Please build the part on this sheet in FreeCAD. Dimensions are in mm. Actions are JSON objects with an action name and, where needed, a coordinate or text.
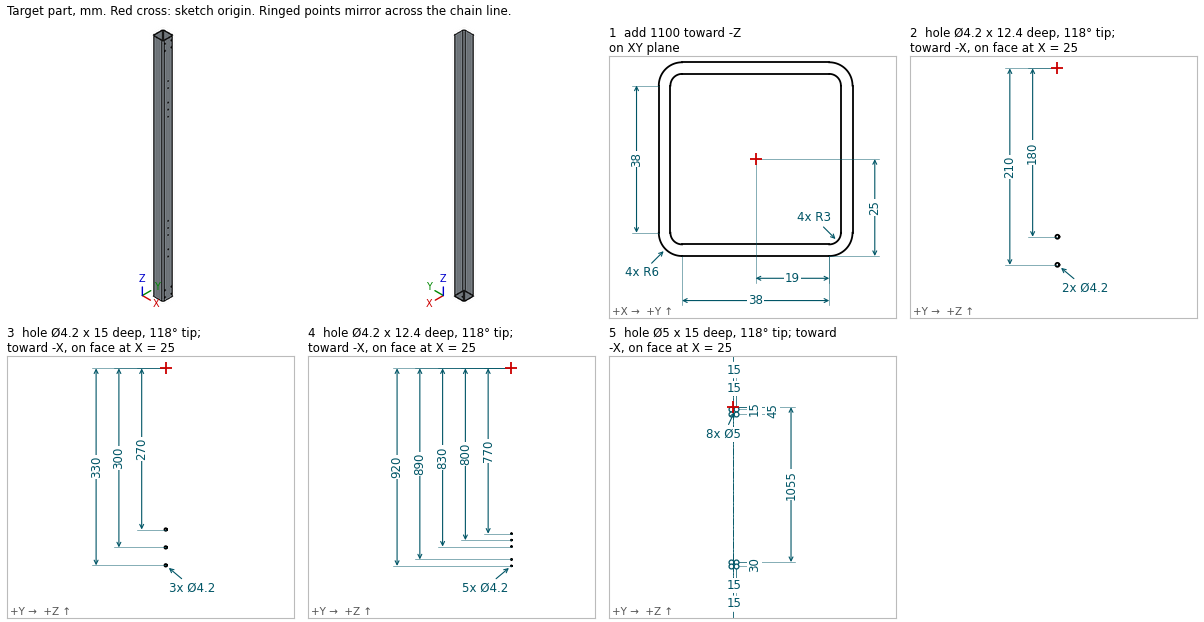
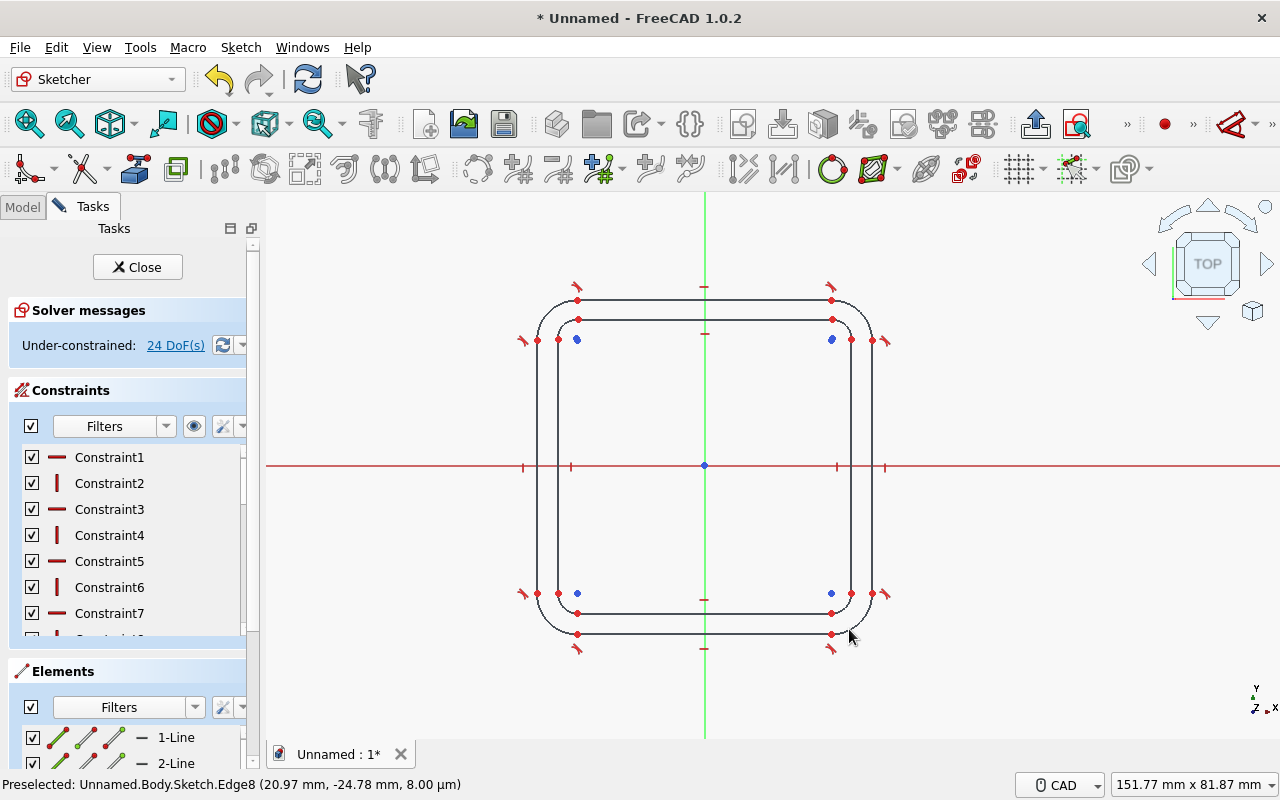
{"action": "left_click", "coordinate": [654, 614]}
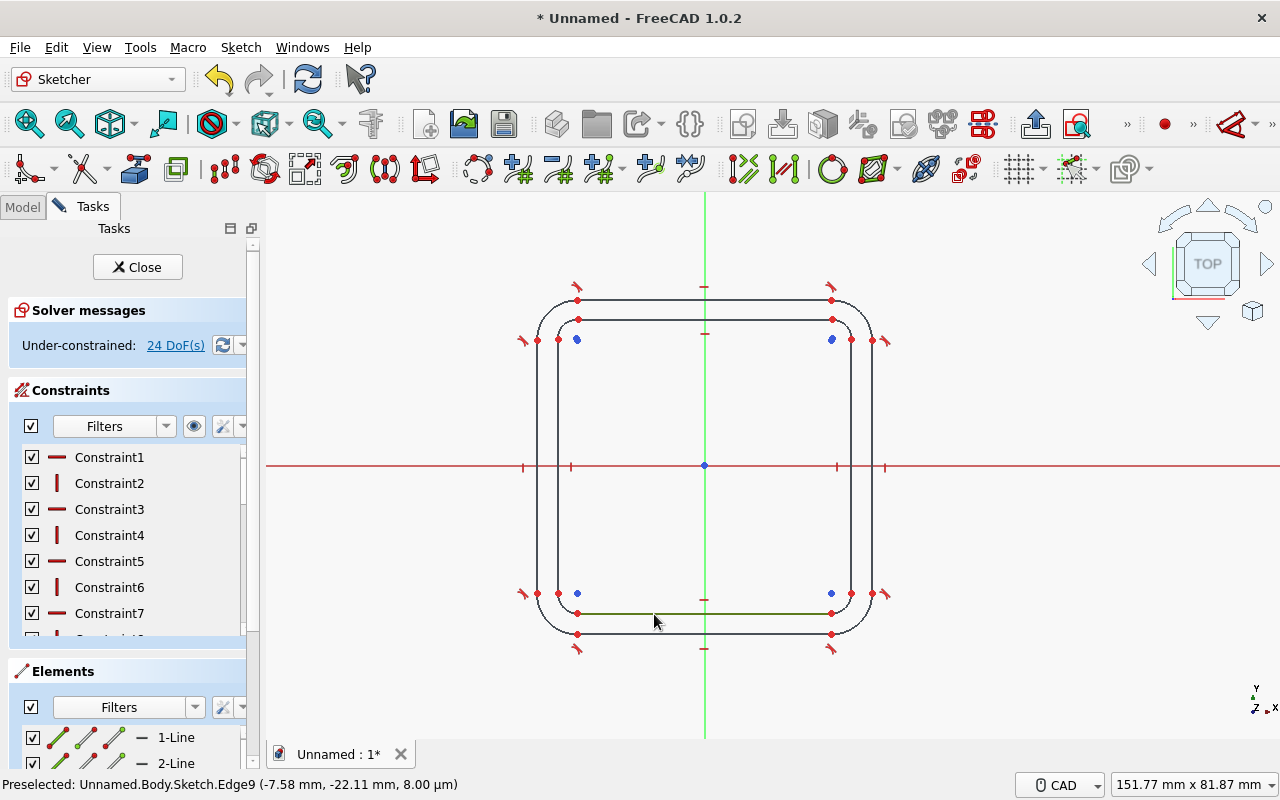
{"action": "scroll", "coordinate": [840, 611], "scroll_direction": "up", "scroll_amount": 2}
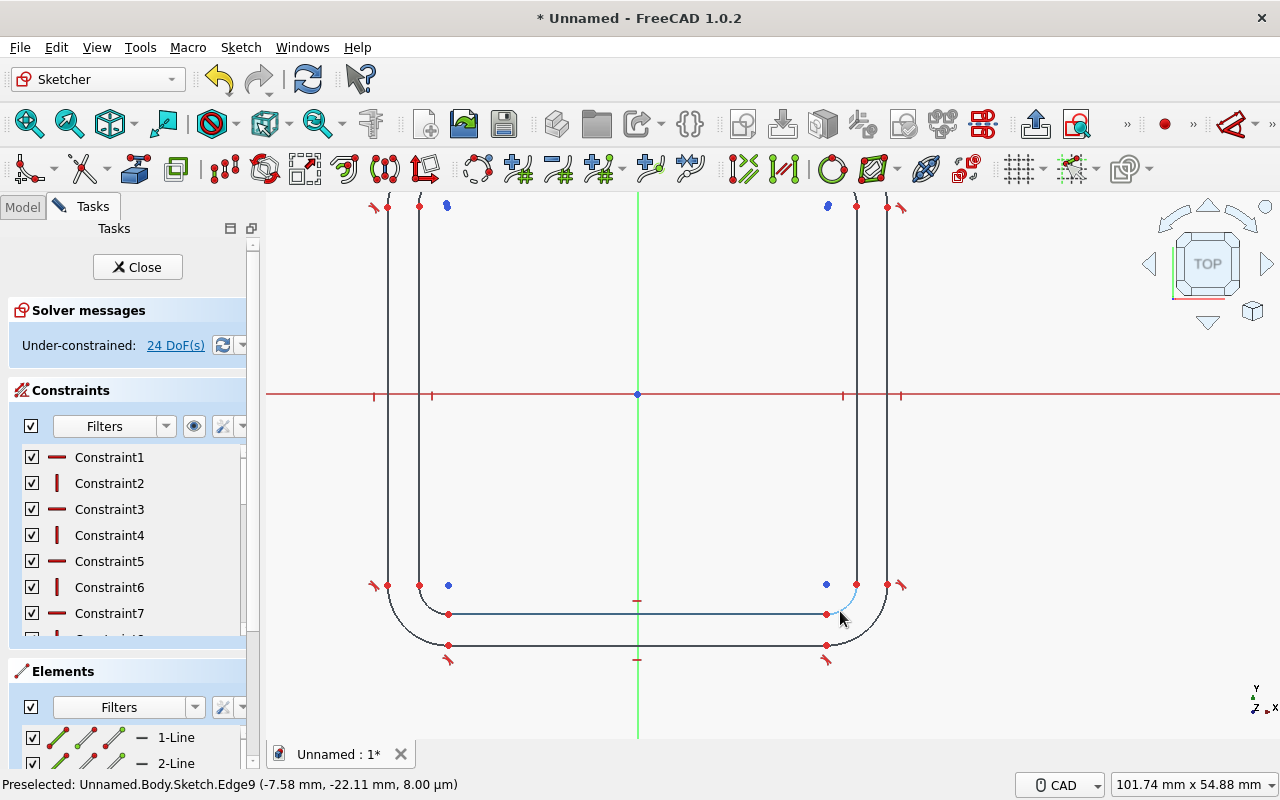
{"action": "left_click", "coordinate": [840, 611]}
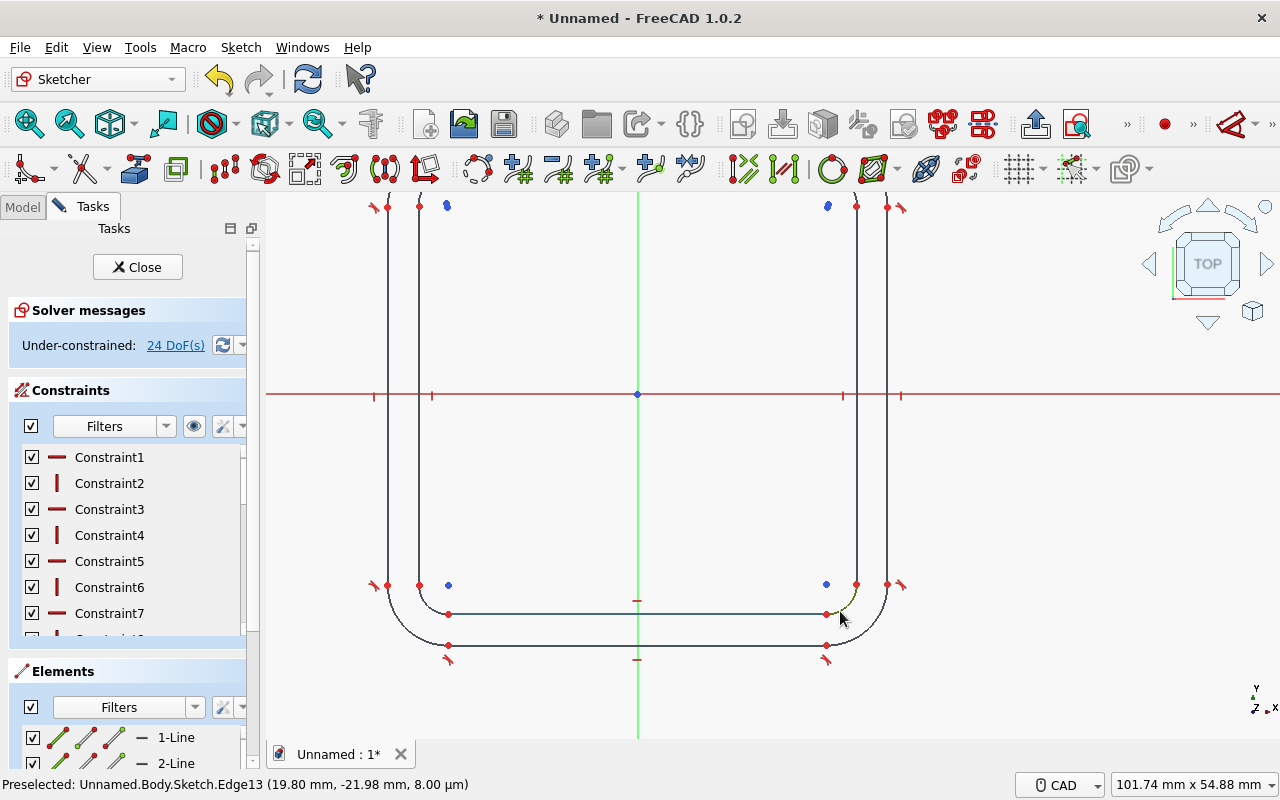
{"action": "key", "text": "t"}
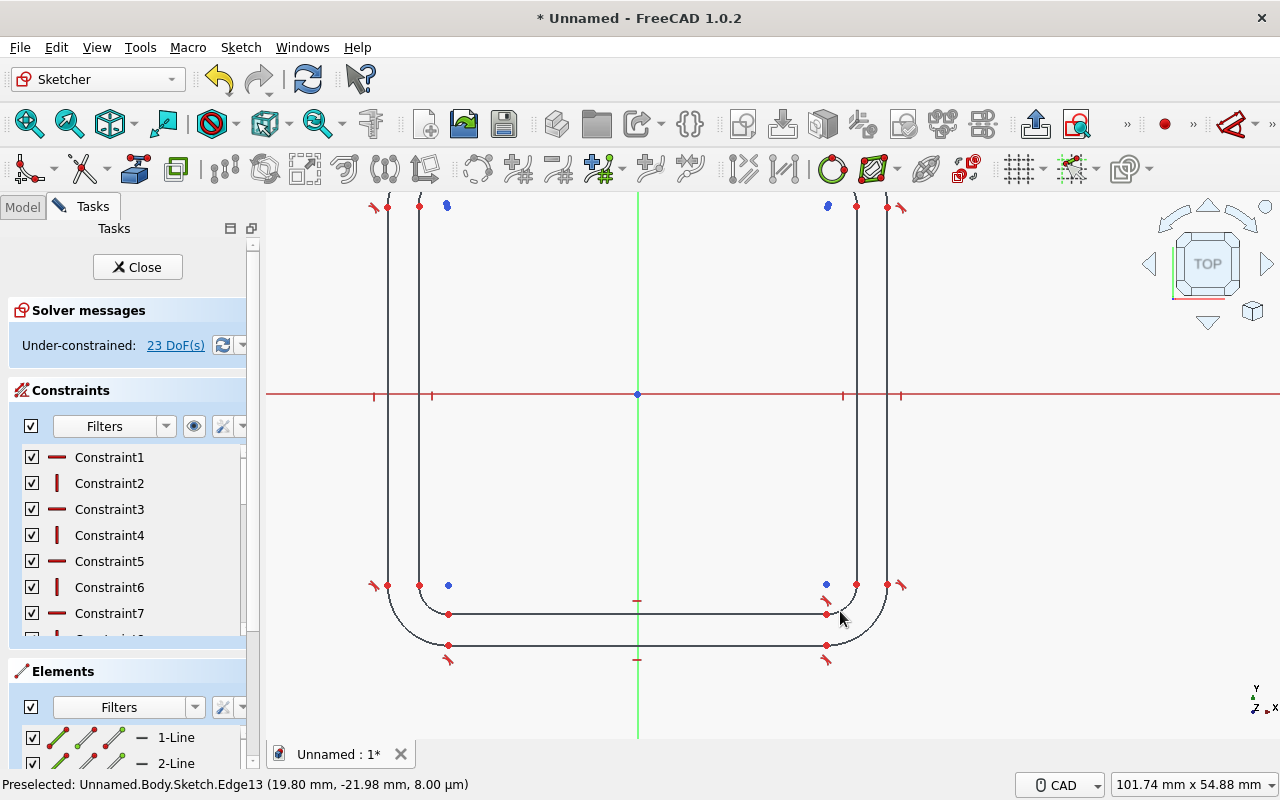
{"action": "left_click", "coordinate": [562, 614]}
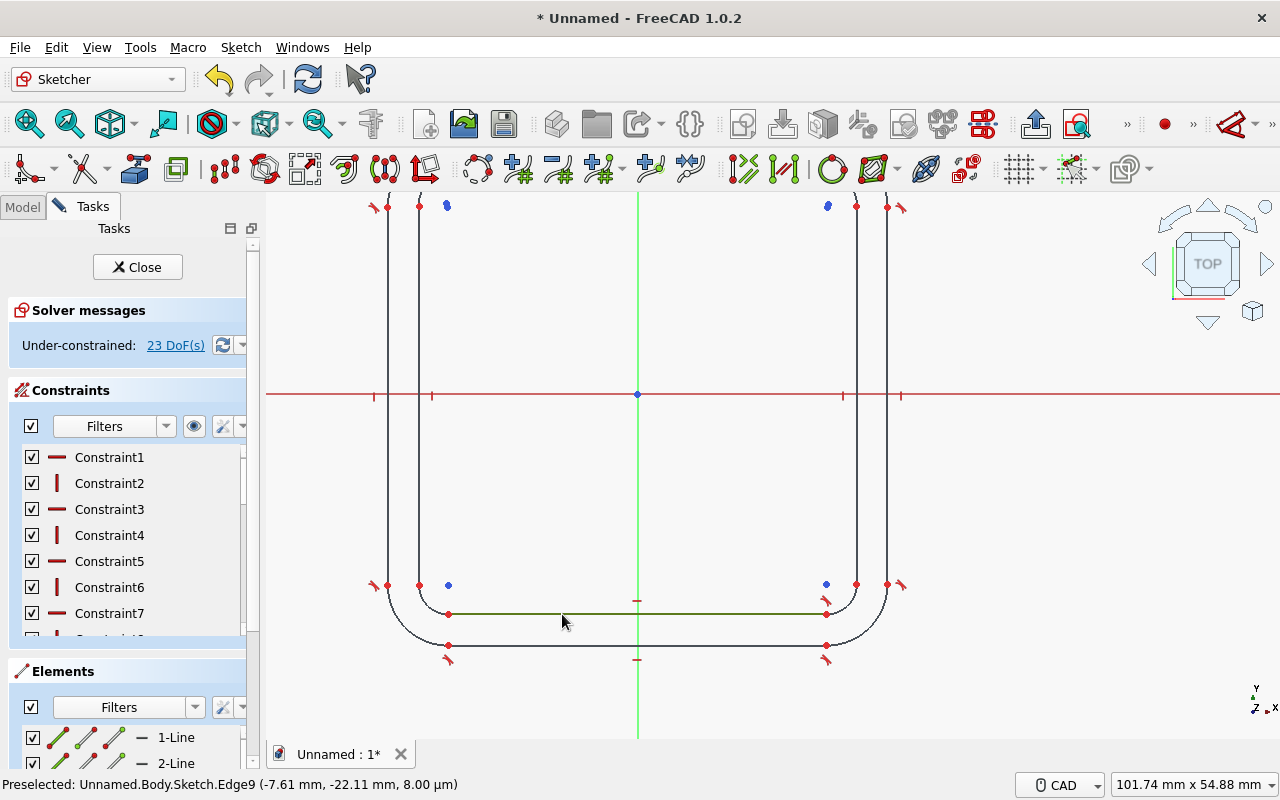
{"action": "left_click", "coordinate": [422, 599]}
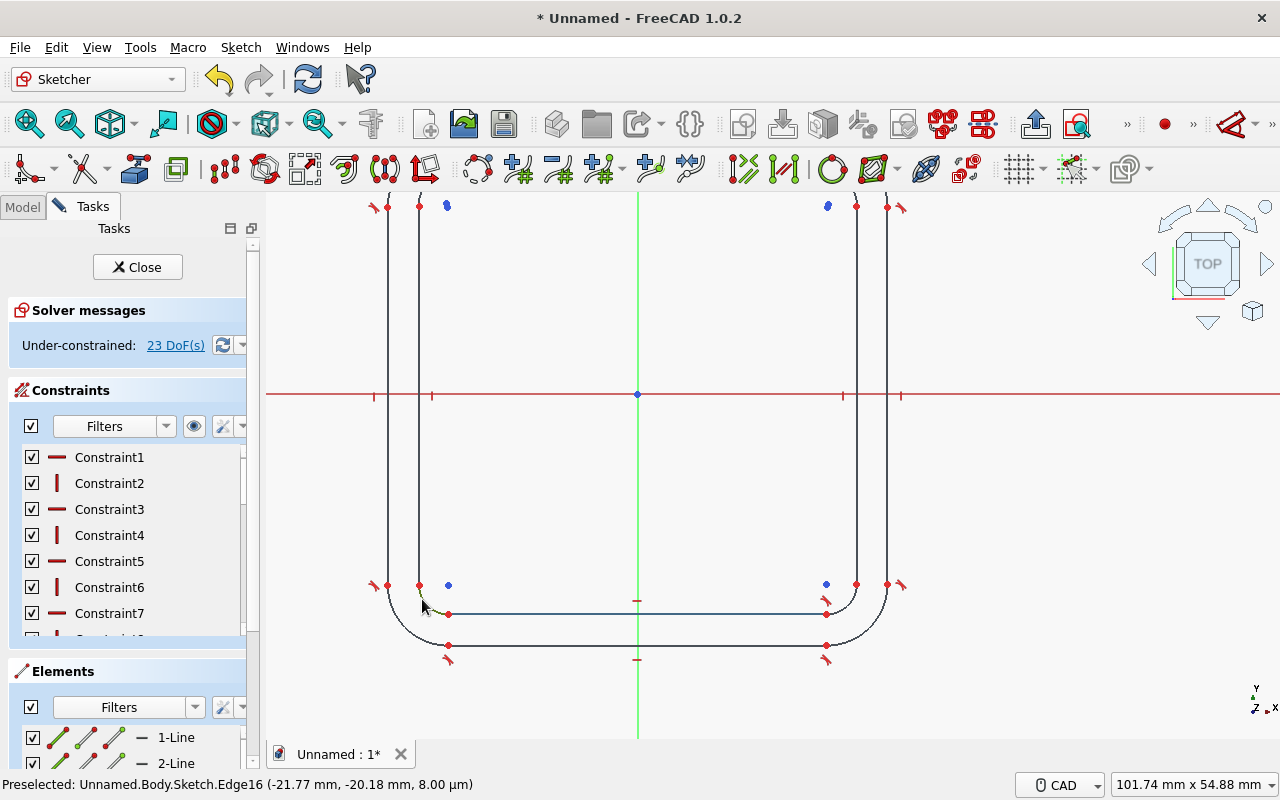
{"action": "key", "text": "t"}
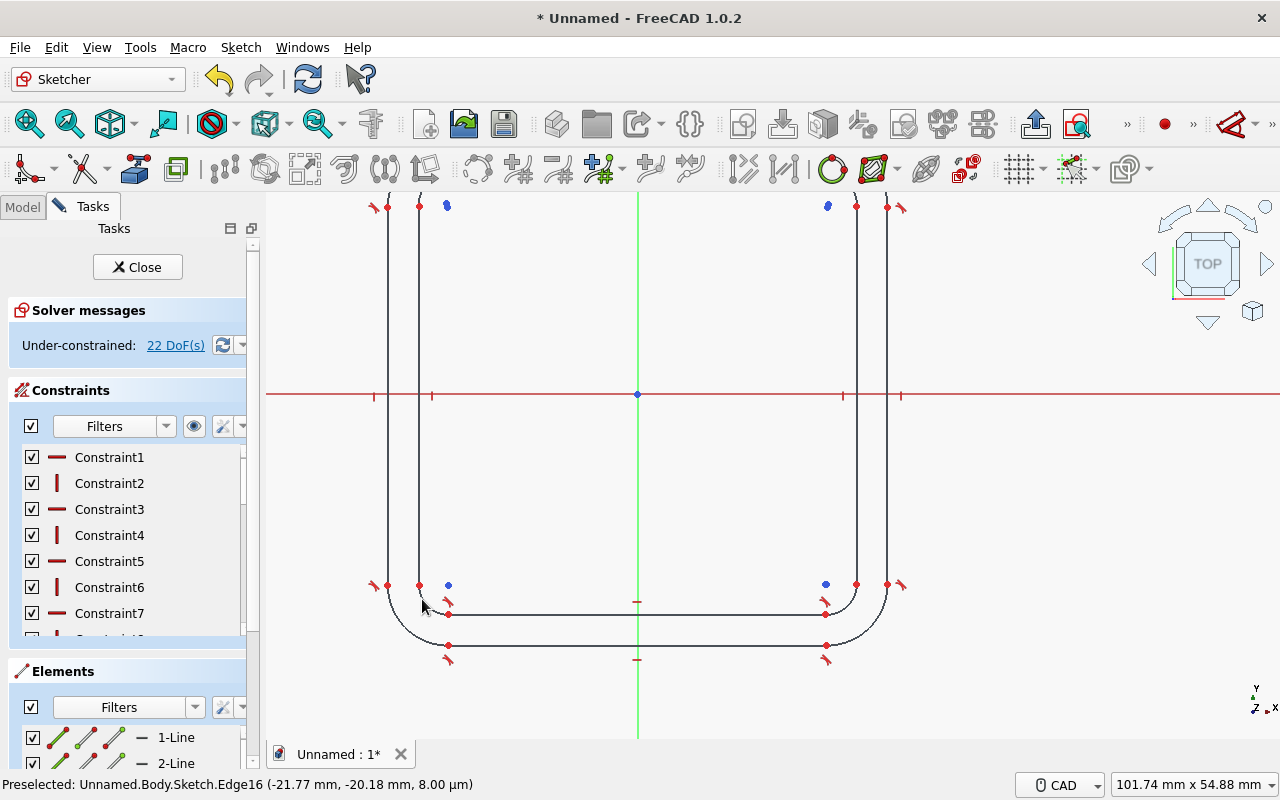
{"action": "left_click", "coordinate": [857, 471]}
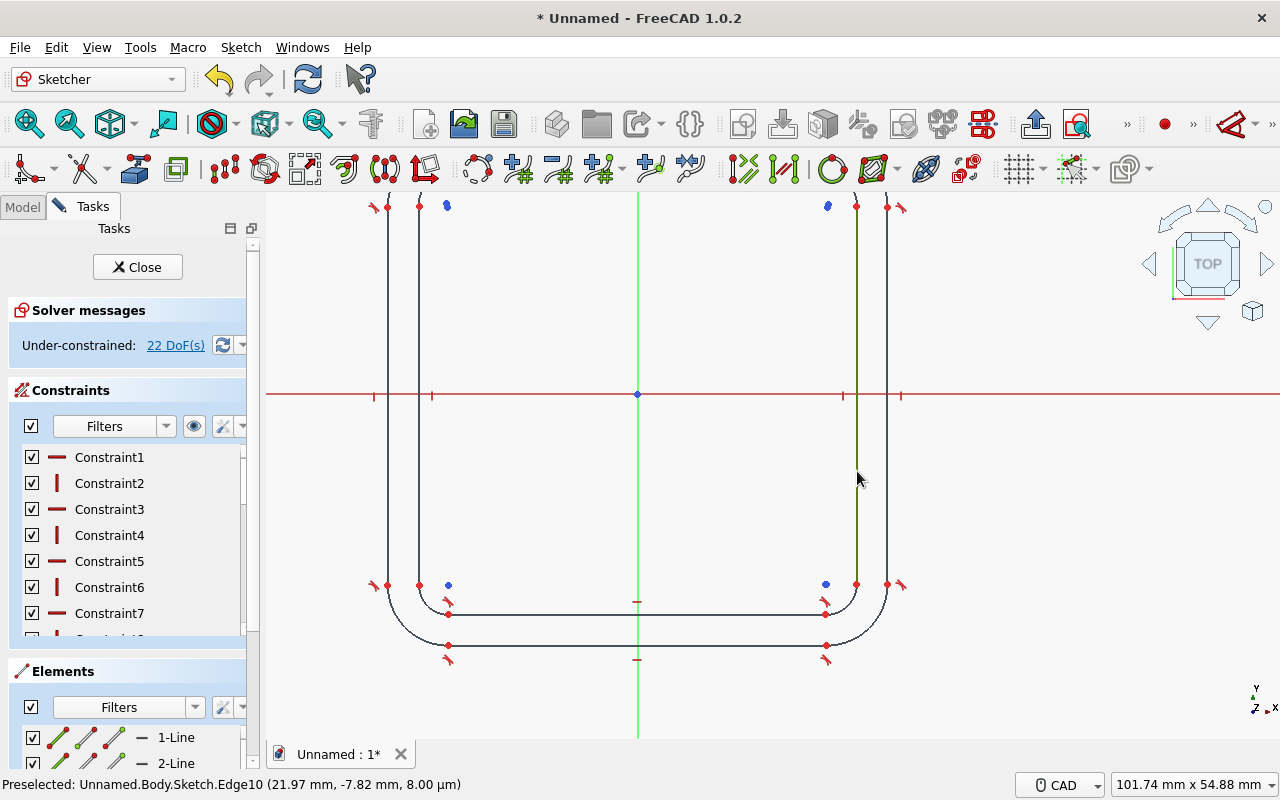
{"action": "left_click", "coordinate": [840, 612]}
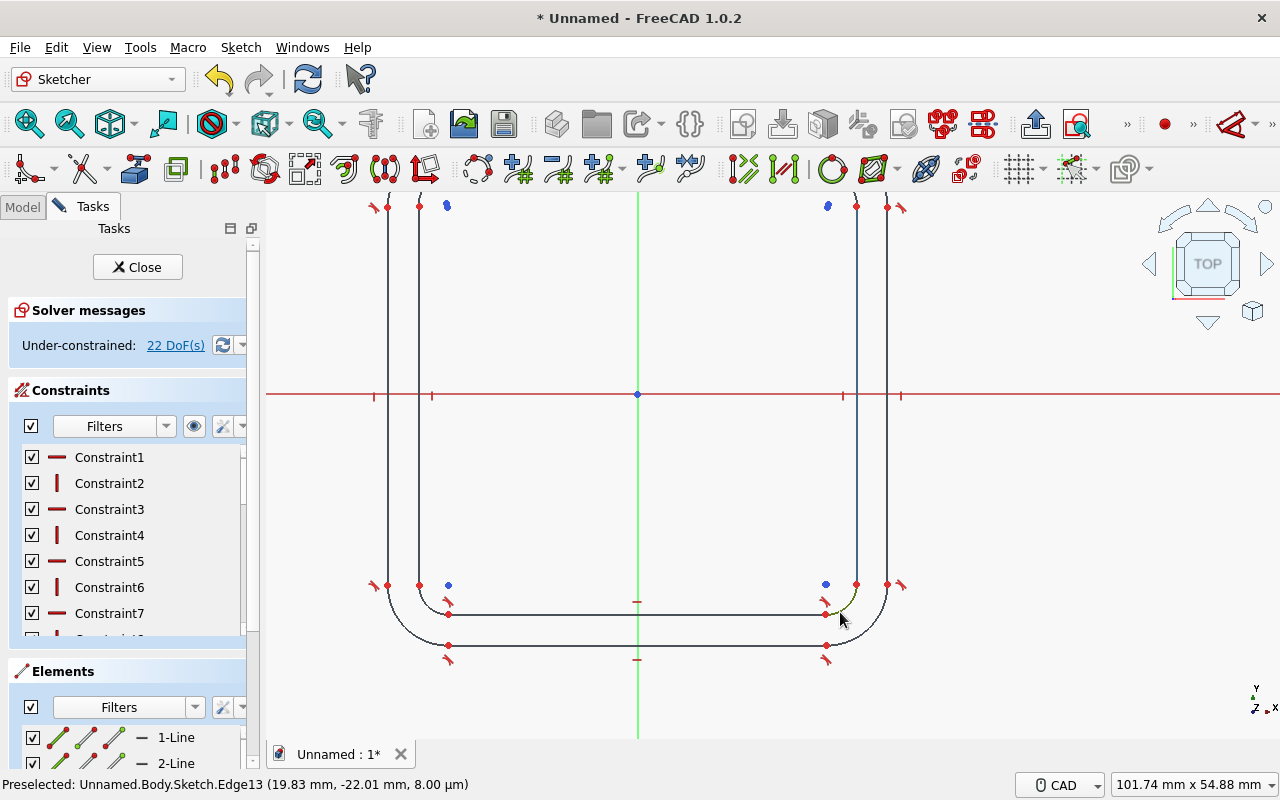
{"action": "key", "text": "t"}